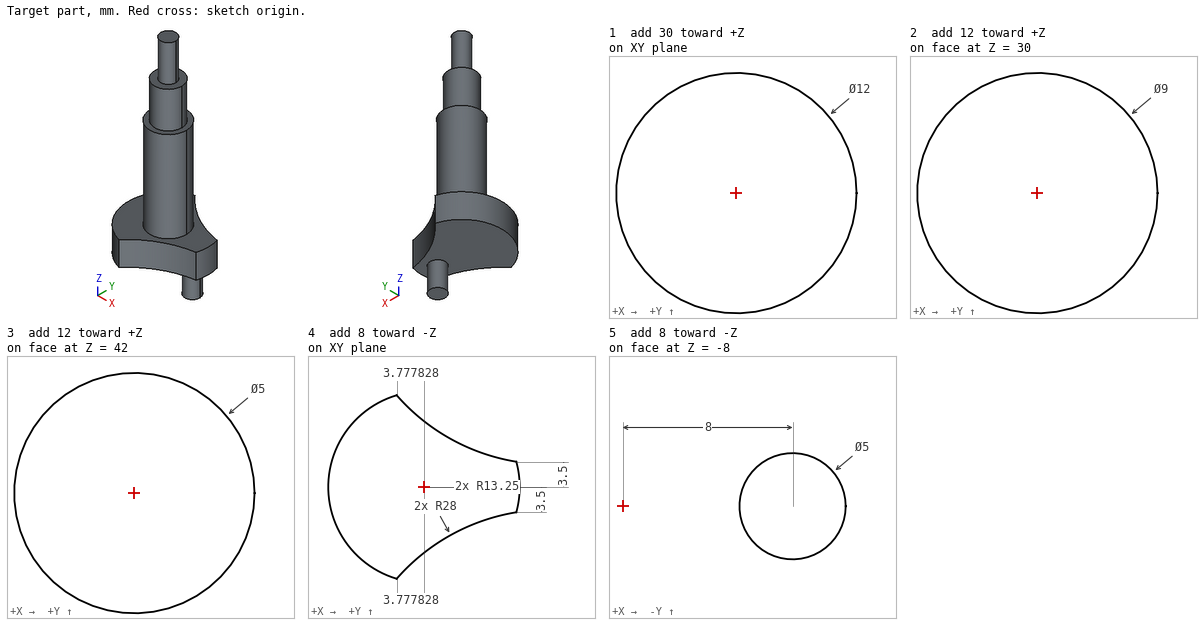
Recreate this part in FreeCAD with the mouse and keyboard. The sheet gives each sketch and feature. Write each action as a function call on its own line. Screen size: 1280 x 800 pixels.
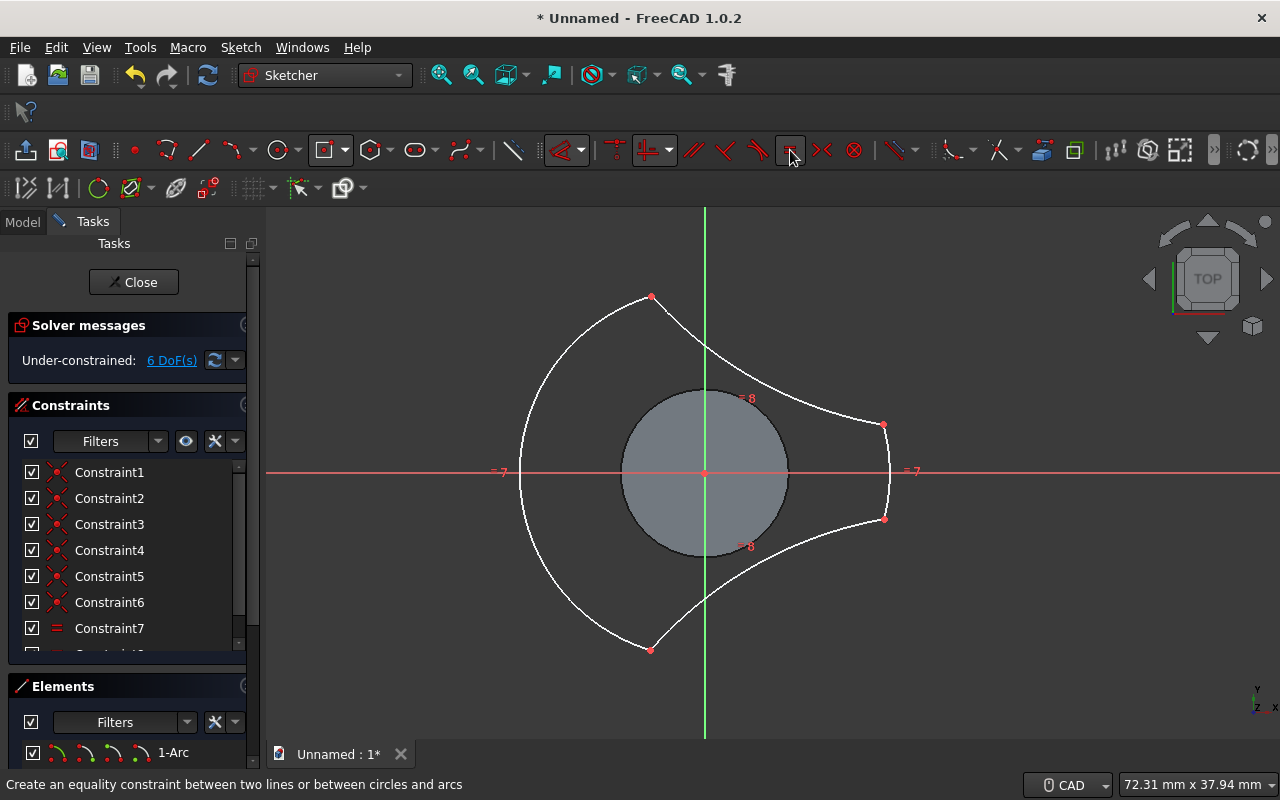
click(560, 150)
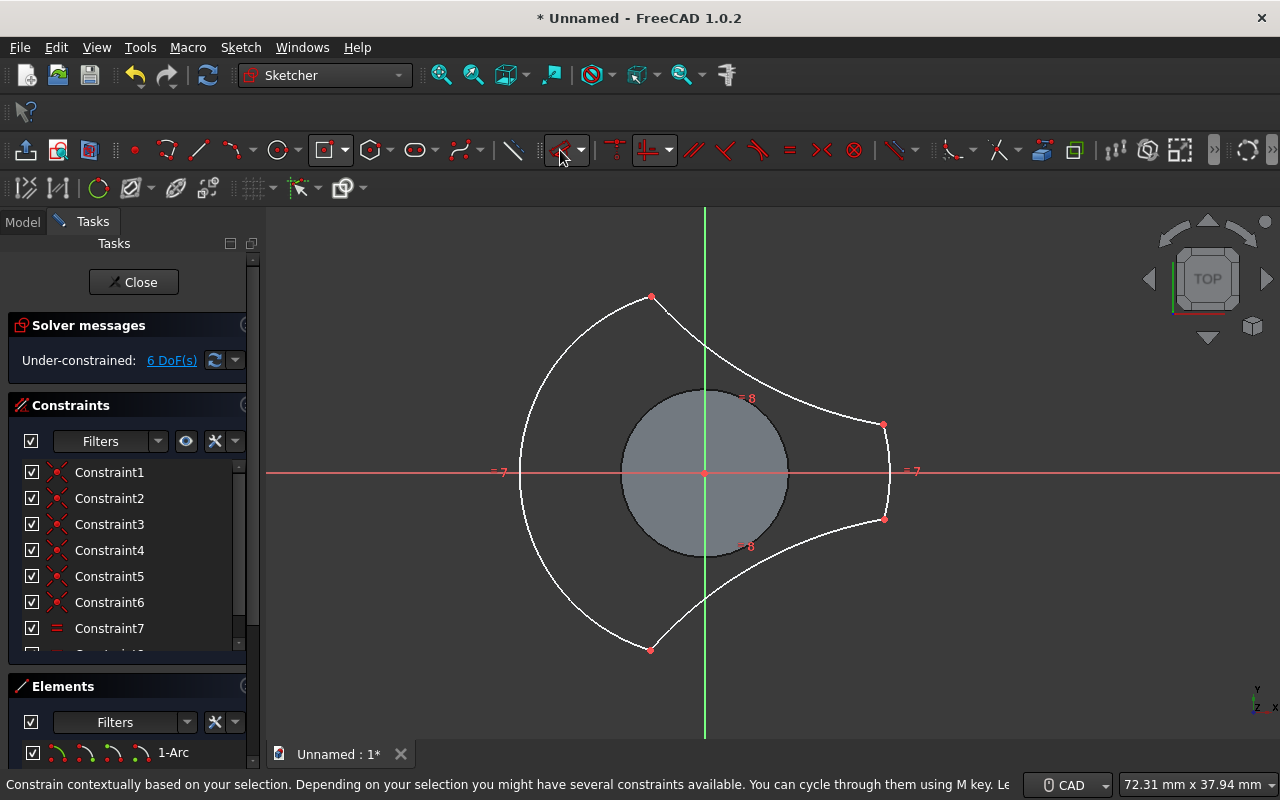
click(544, 382)
click(516, 366)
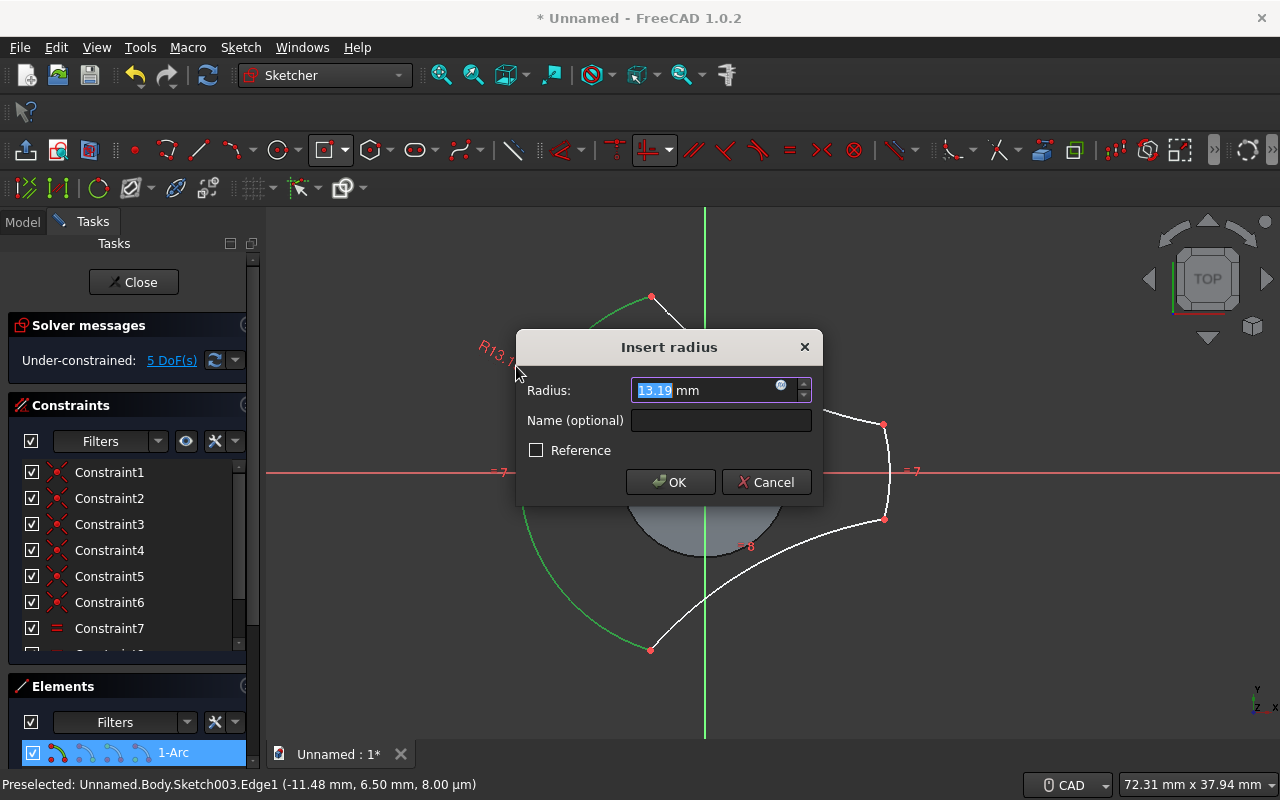
text(13.25)
key(Return)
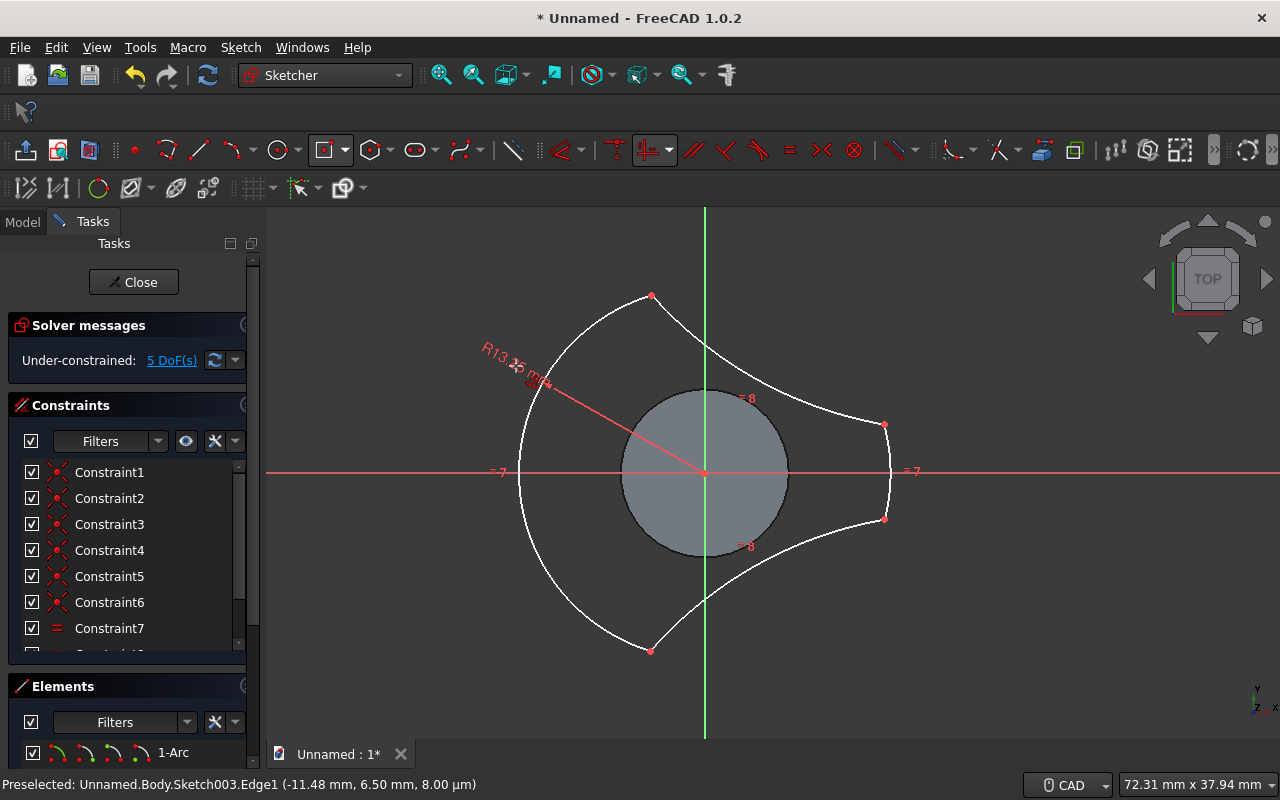
click(806, 403)
click(794, 433)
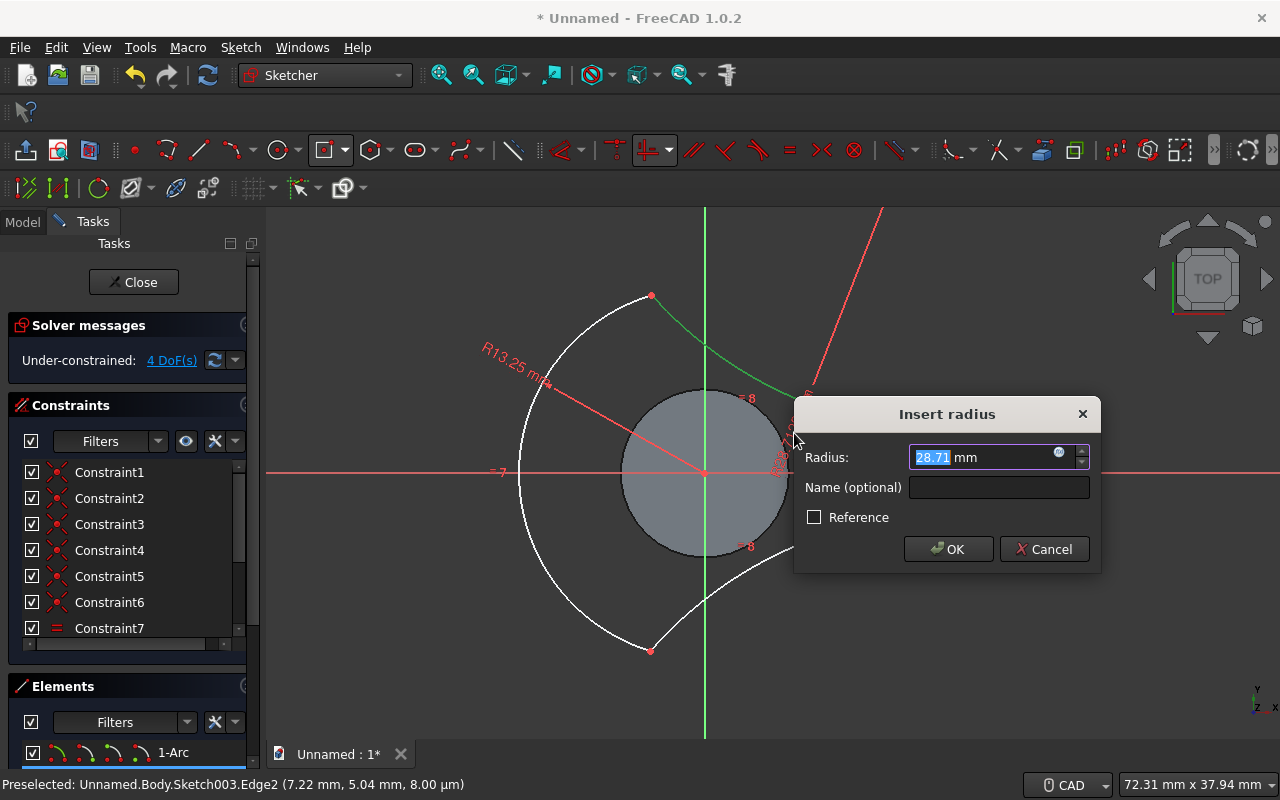
text(28)
key(Return)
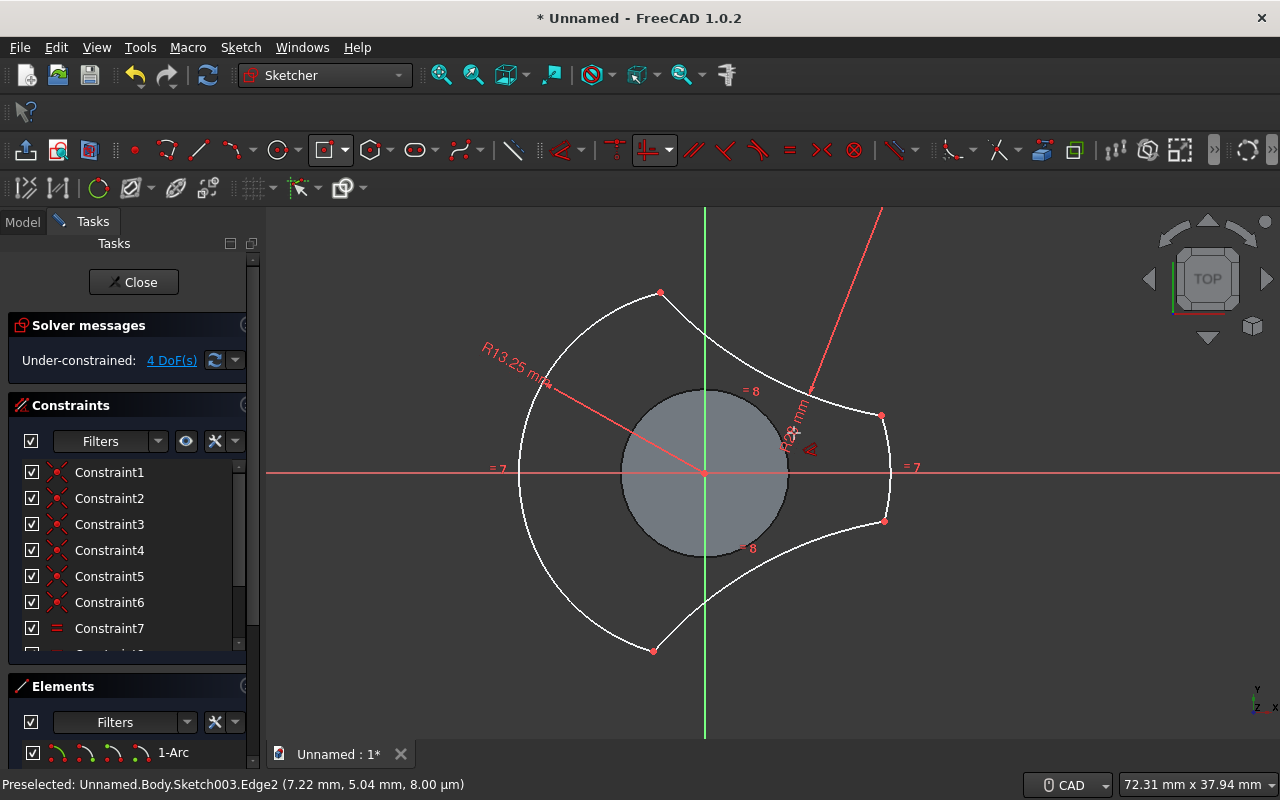
click(881, 416)
click(915, 445)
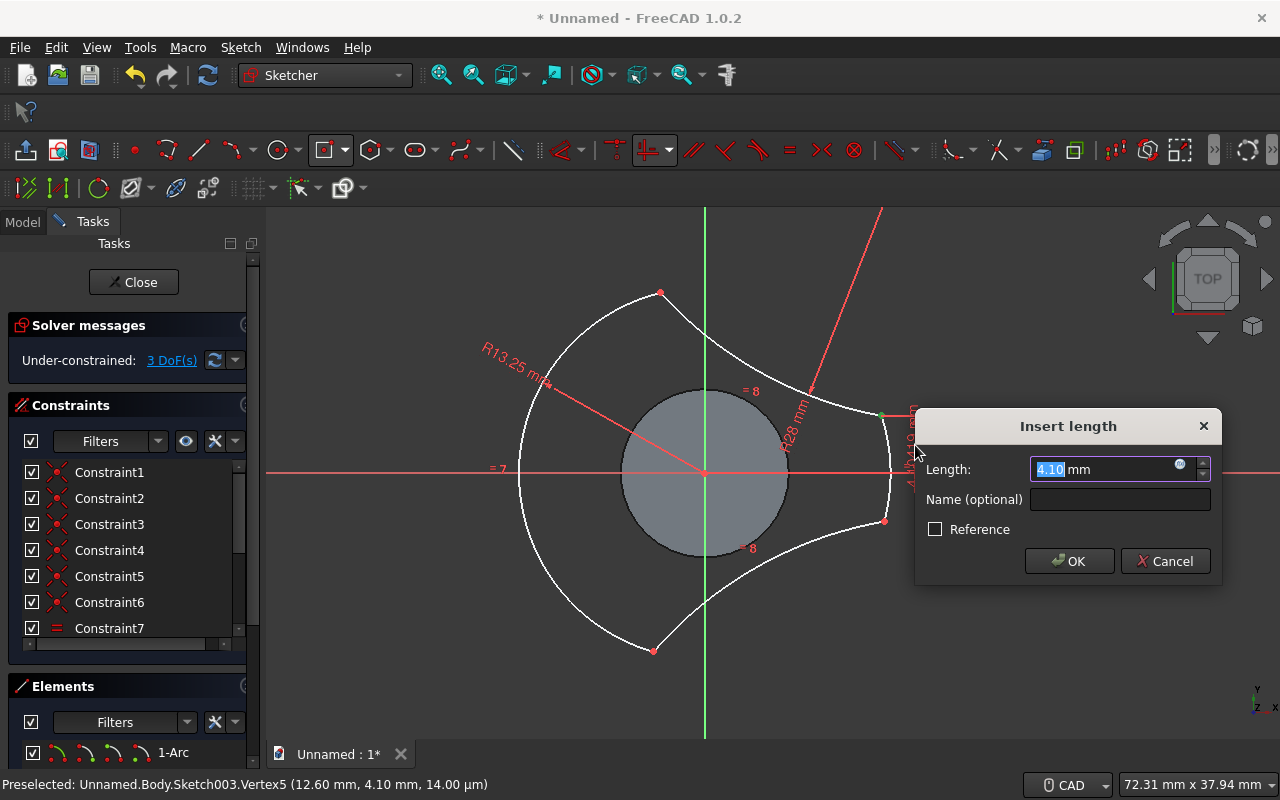
text(3.5)
key(Return)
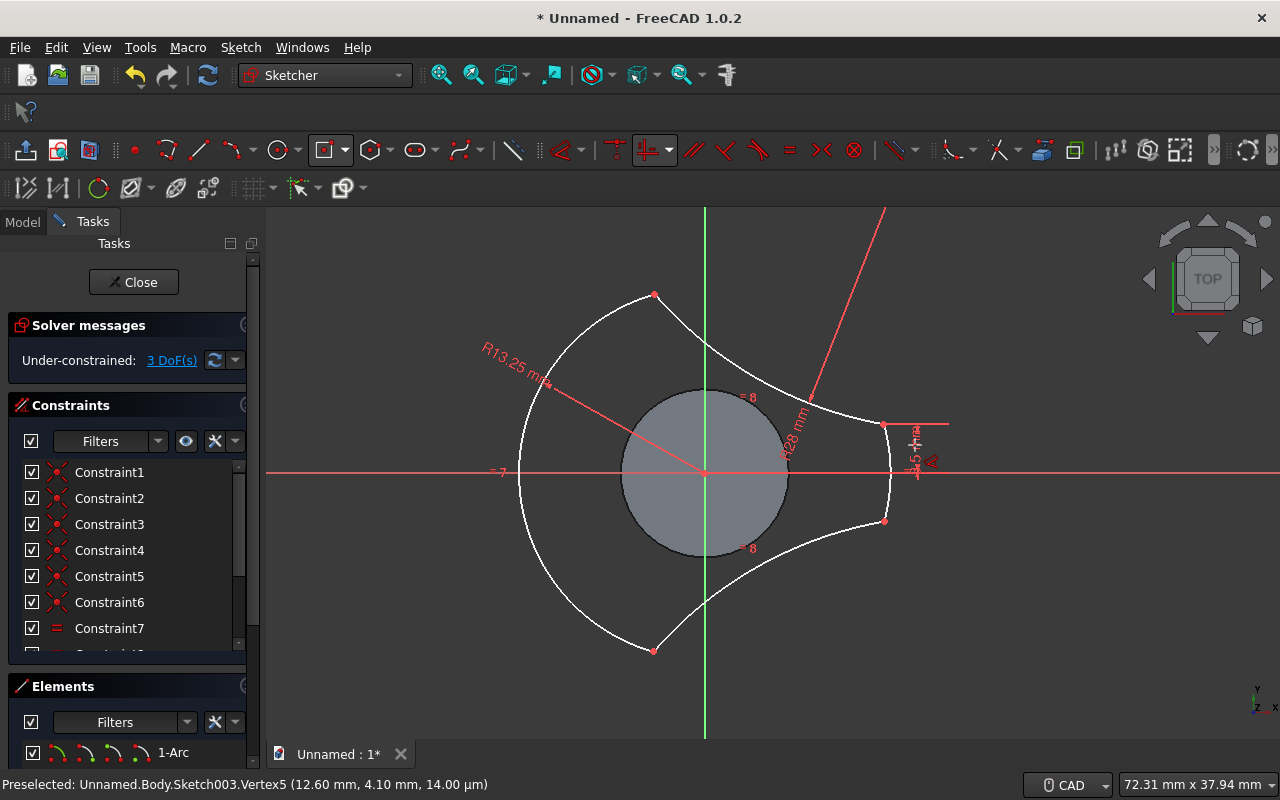
click(884, 522)
click(918, 498)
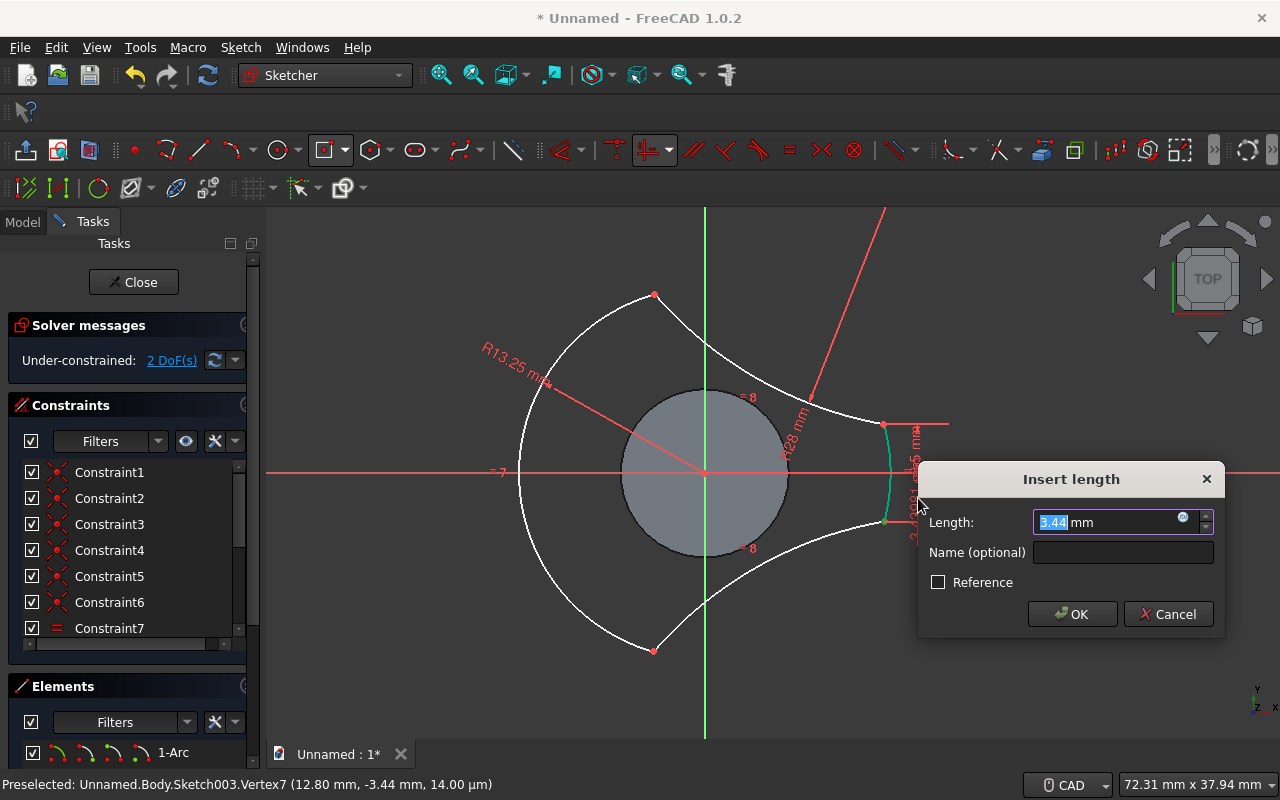
text(3.5)
key(Return)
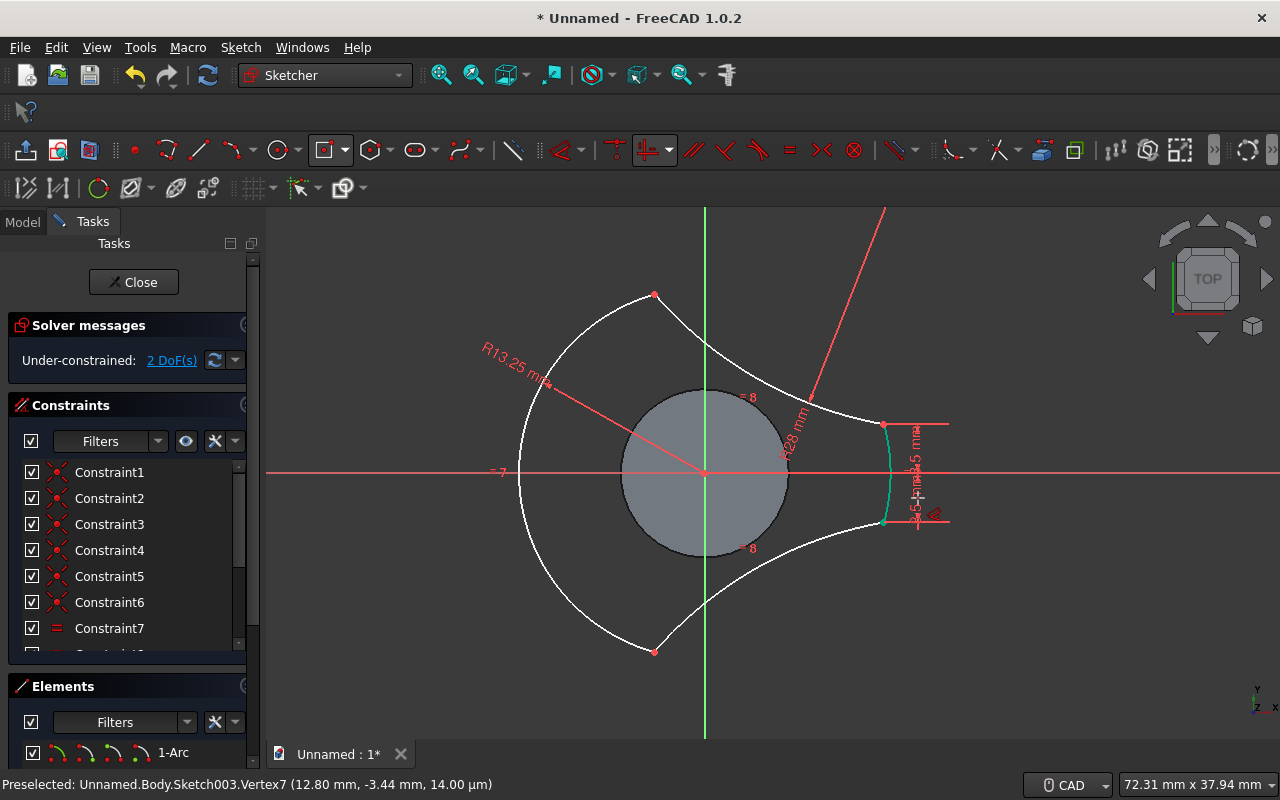
click(655, 294)
click(680, 260)